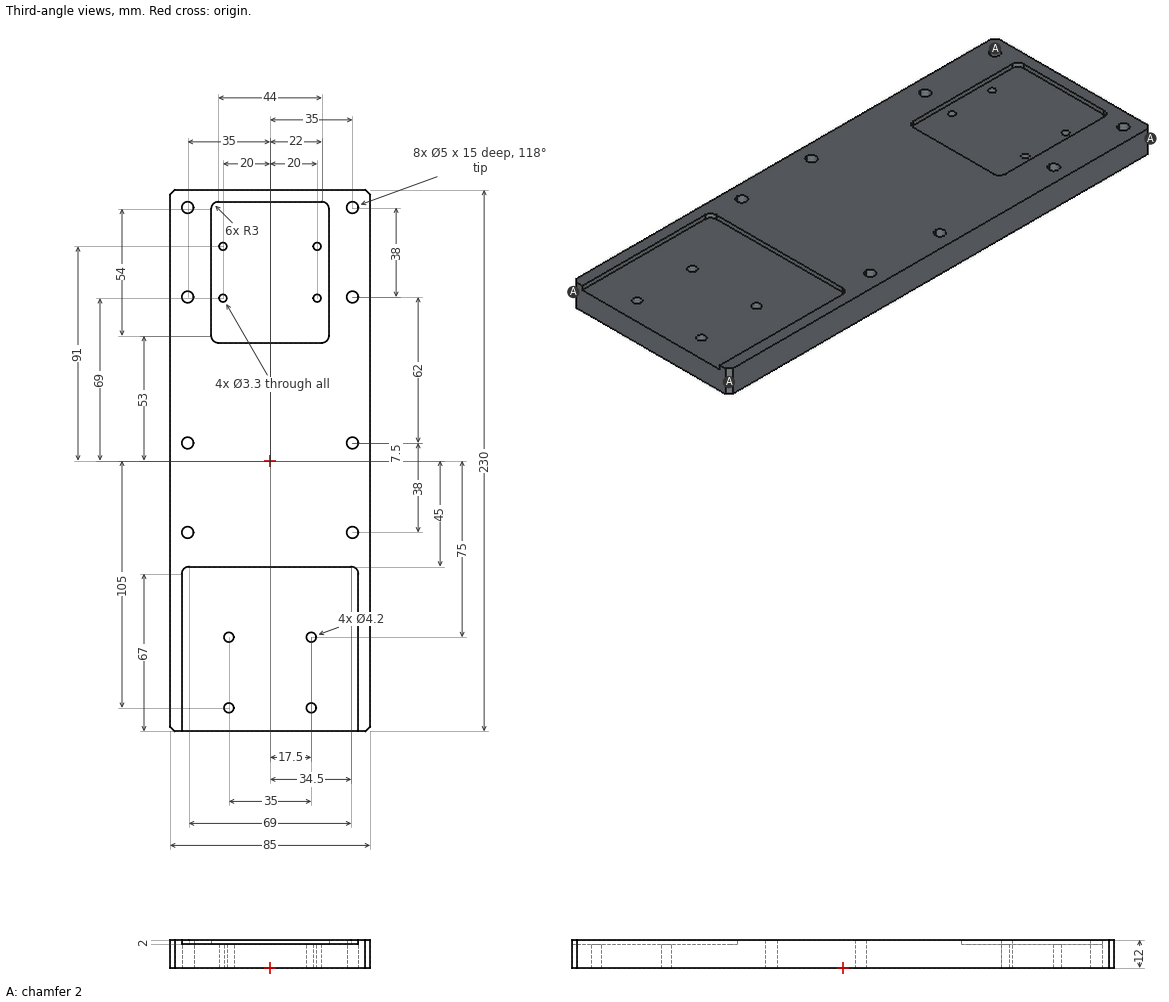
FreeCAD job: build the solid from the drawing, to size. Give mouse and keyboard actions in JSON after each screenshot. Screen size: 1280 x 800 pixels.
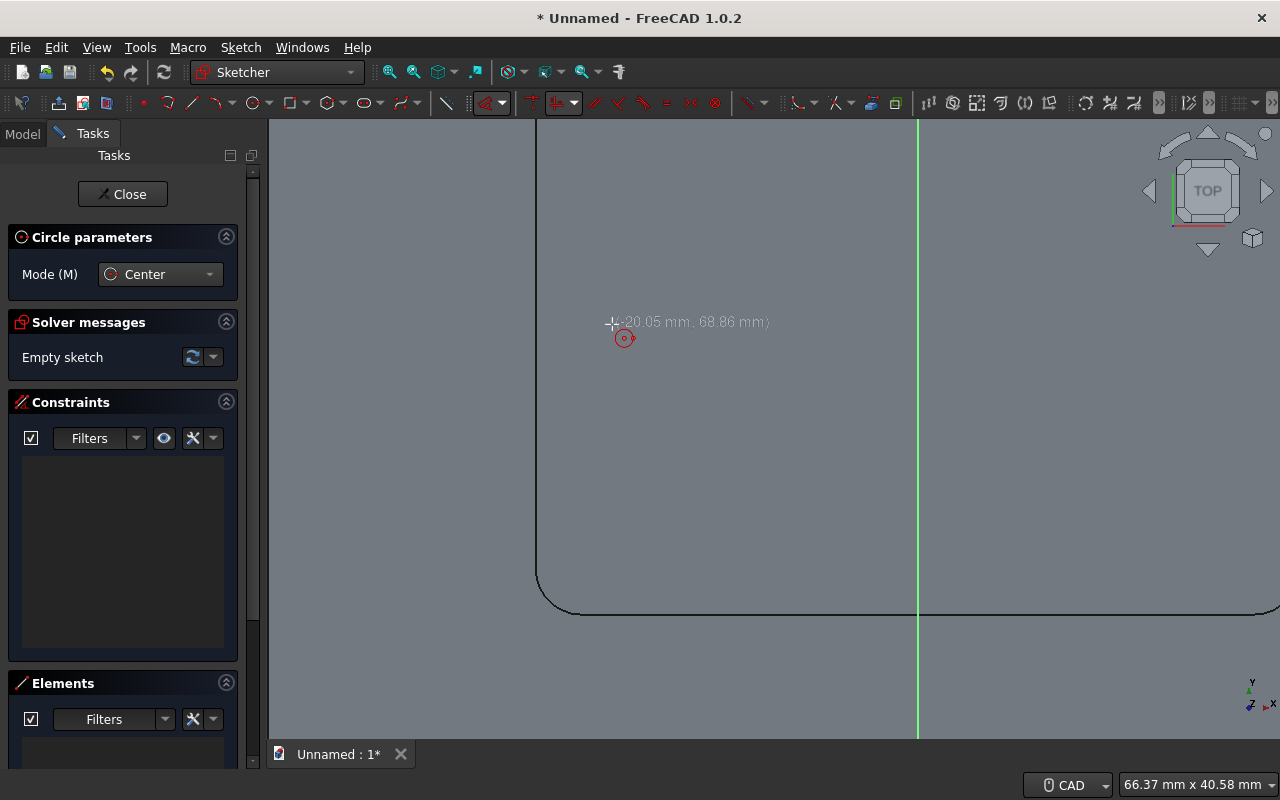
{"action": "left_click", "coordinate": [612, 324]}
{"action": "left_click", "coordinate": [630, 307]}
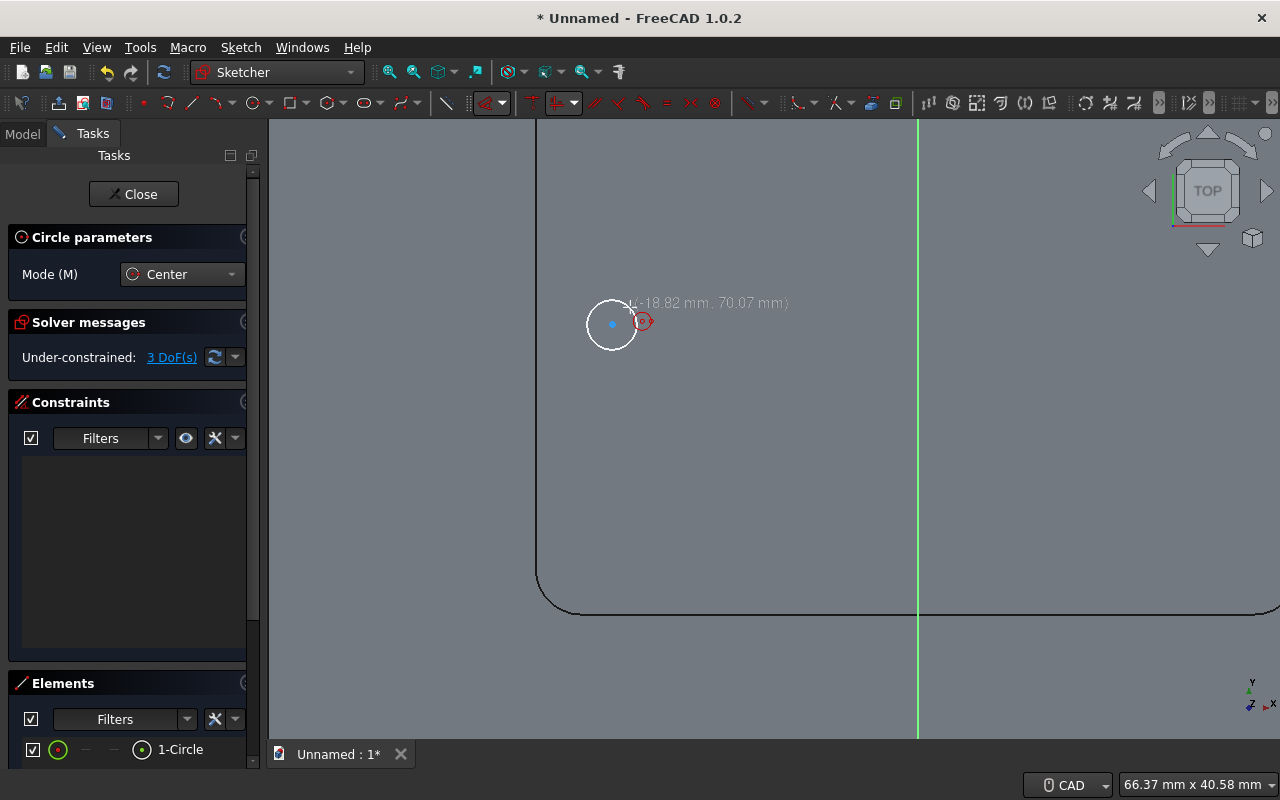
{"action": "scroll", "coordinate": [613, 325], "scroll_direction": "down", "scroll_amount": 6}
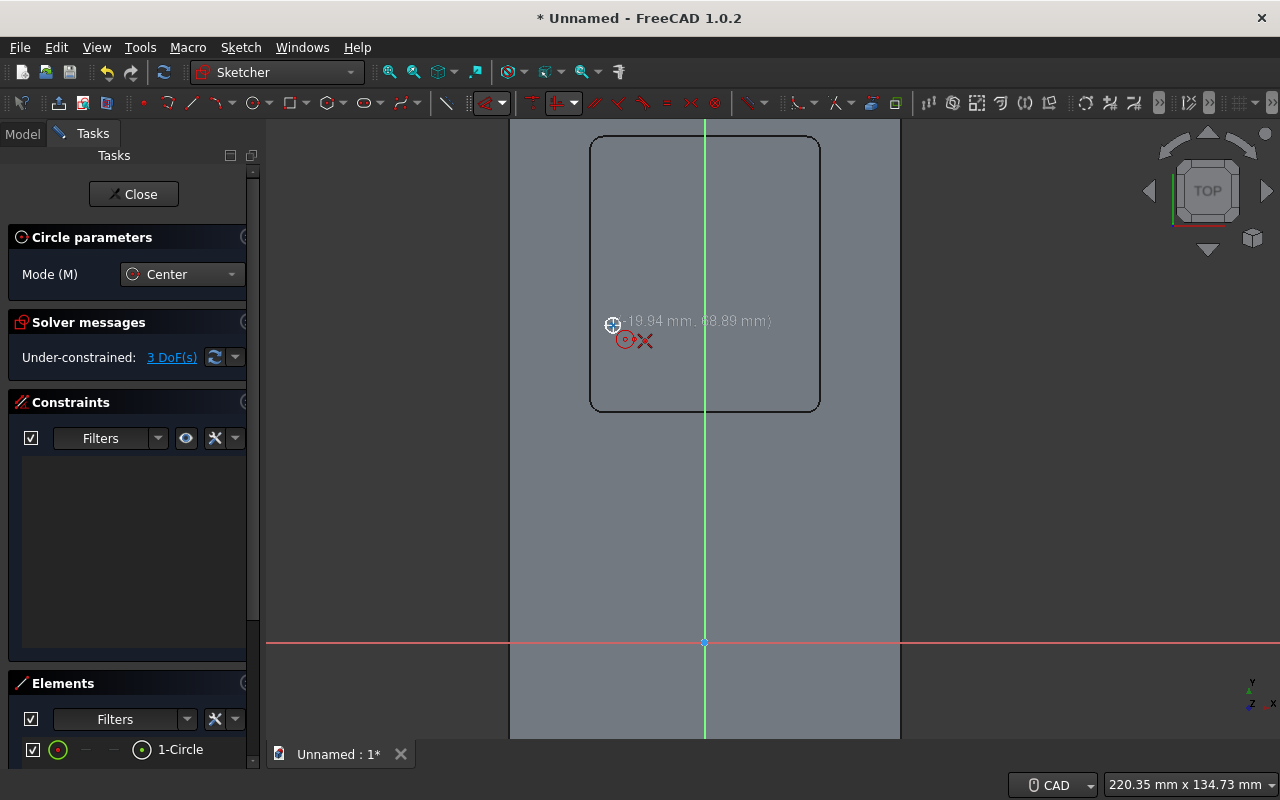
{"action": "scroll", "coordinate": [797, 325], "scroll_direction": "up", "scroll_amount": 6}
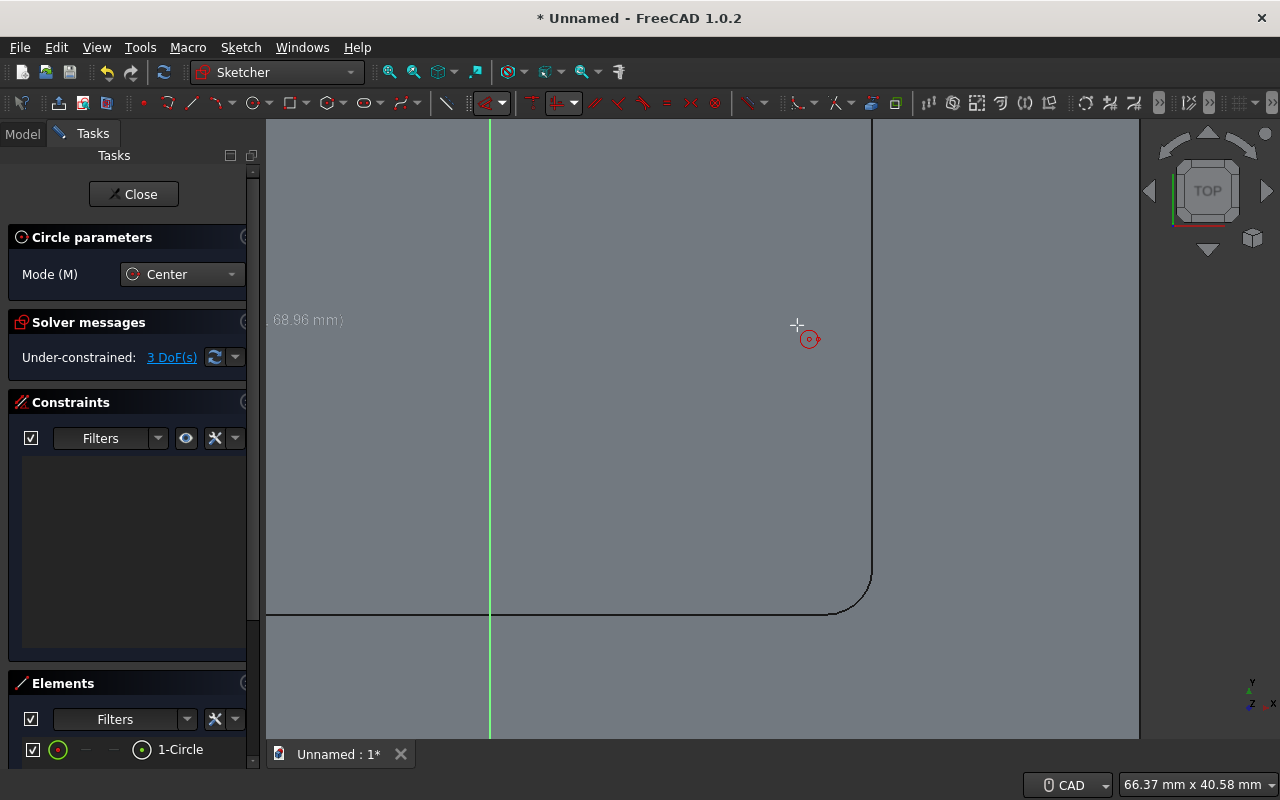
{"action": "left_click", "coordinate": [796, 324]}
{"action": "left_click", "coordinate": [814, 307]}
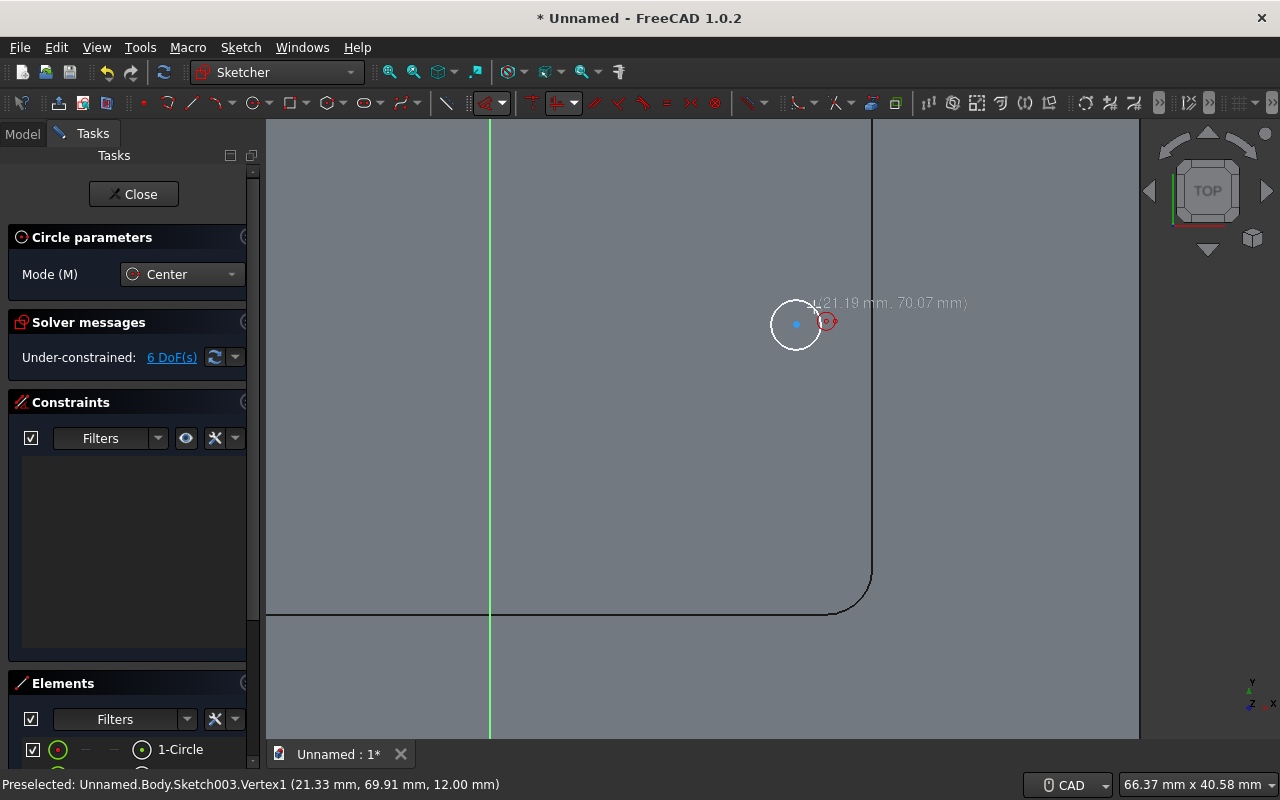
{"action": "scroll", "coordinate": [797, 325], "scroll_direction": "down", "scroll_amount": 6}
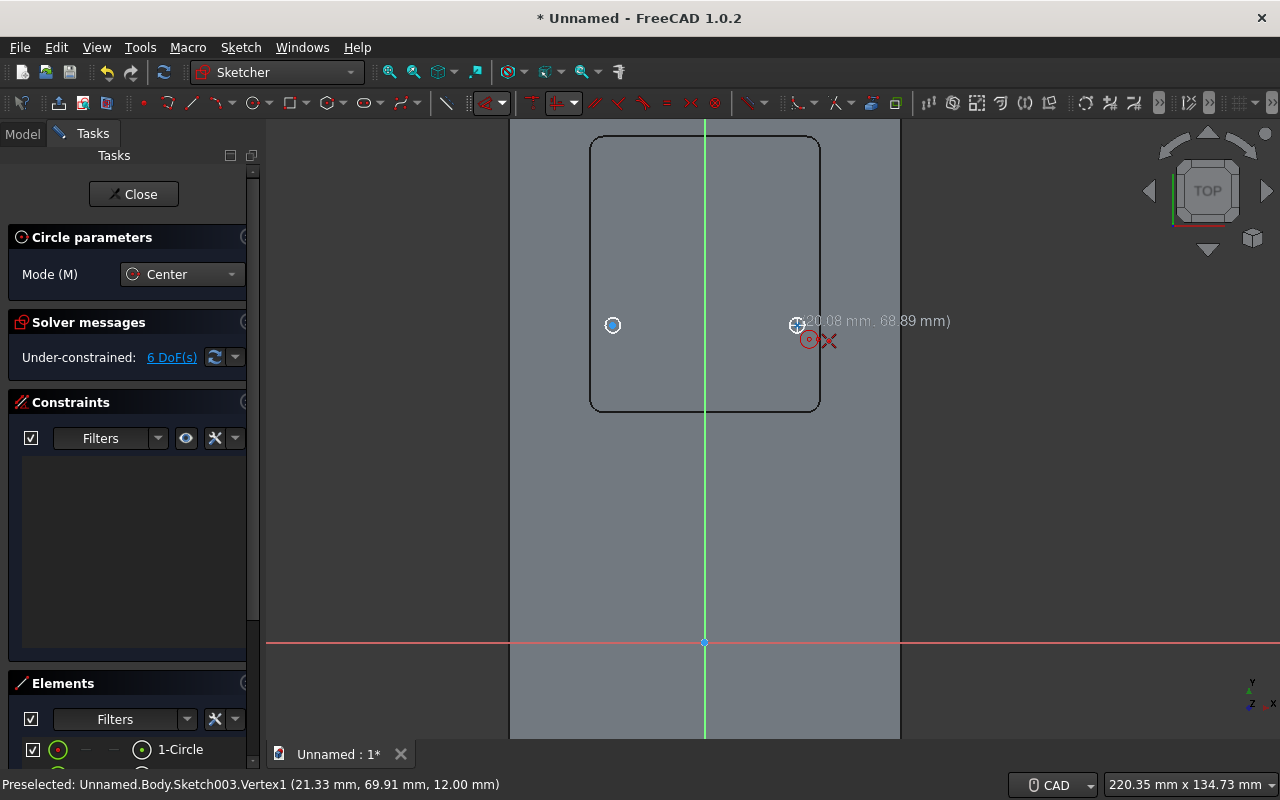
{"action": "scroll", "coordinate": [613, 224], "scroll_direction": "up", "scroll_amount": 6}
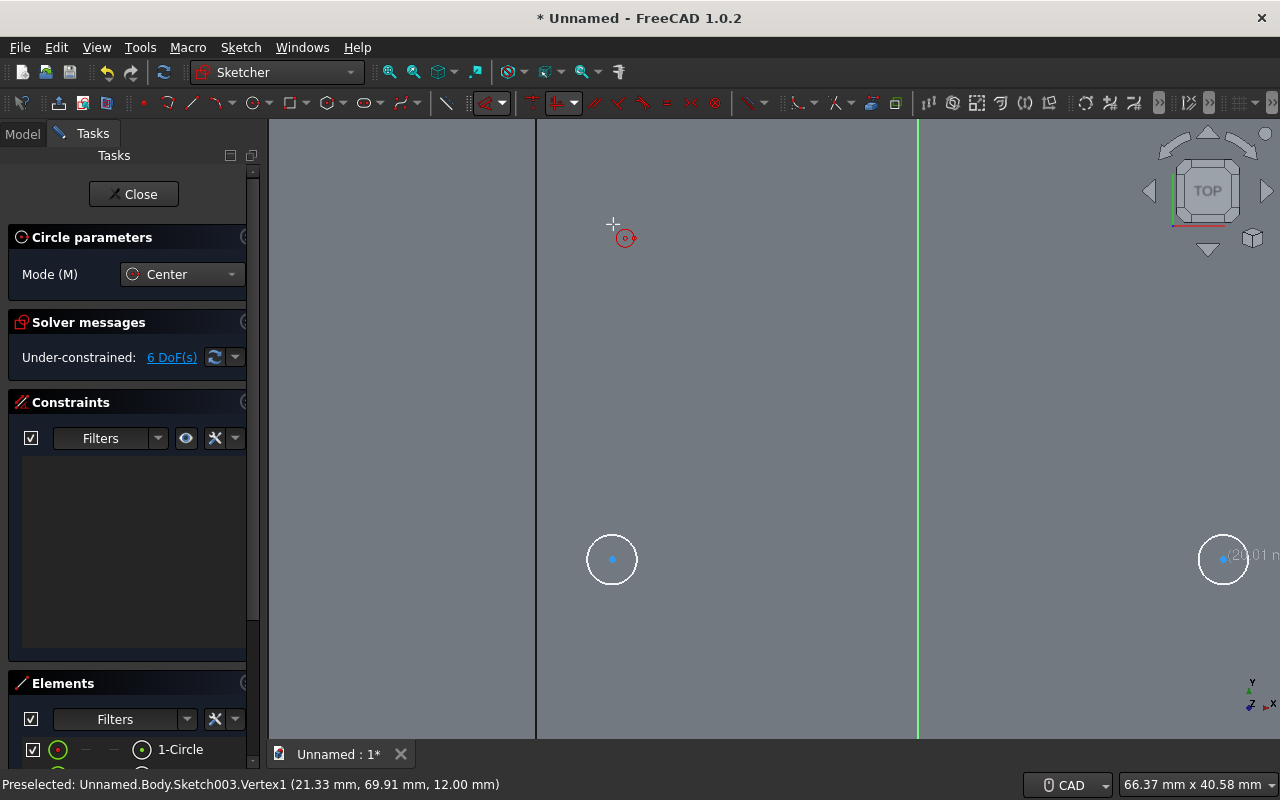
{"action": "left_click", "coordinate": [612, 223]}
{"action": "left_click", "coordinate": [630, 205]}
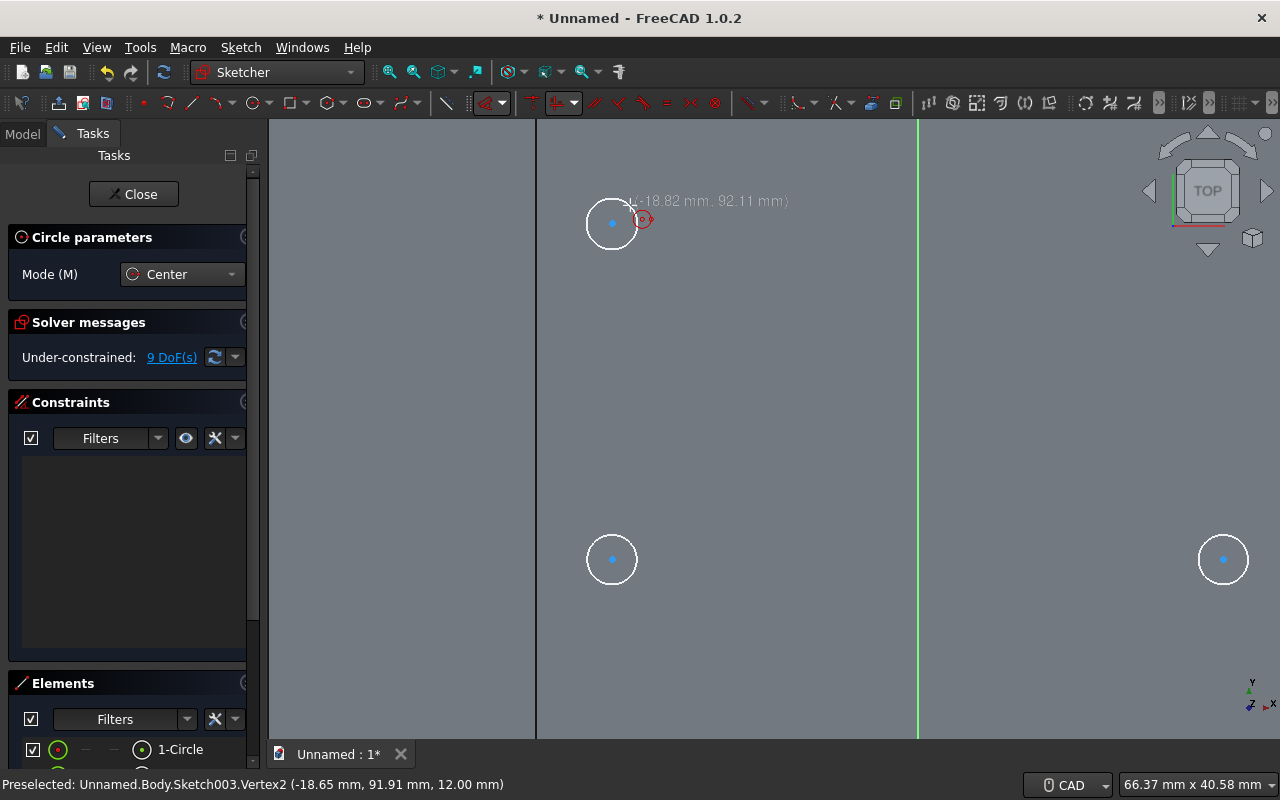
{"action": "scroll", "coordinate": [613, 224], "scroll_direction": "down", "scroll_amount": 6}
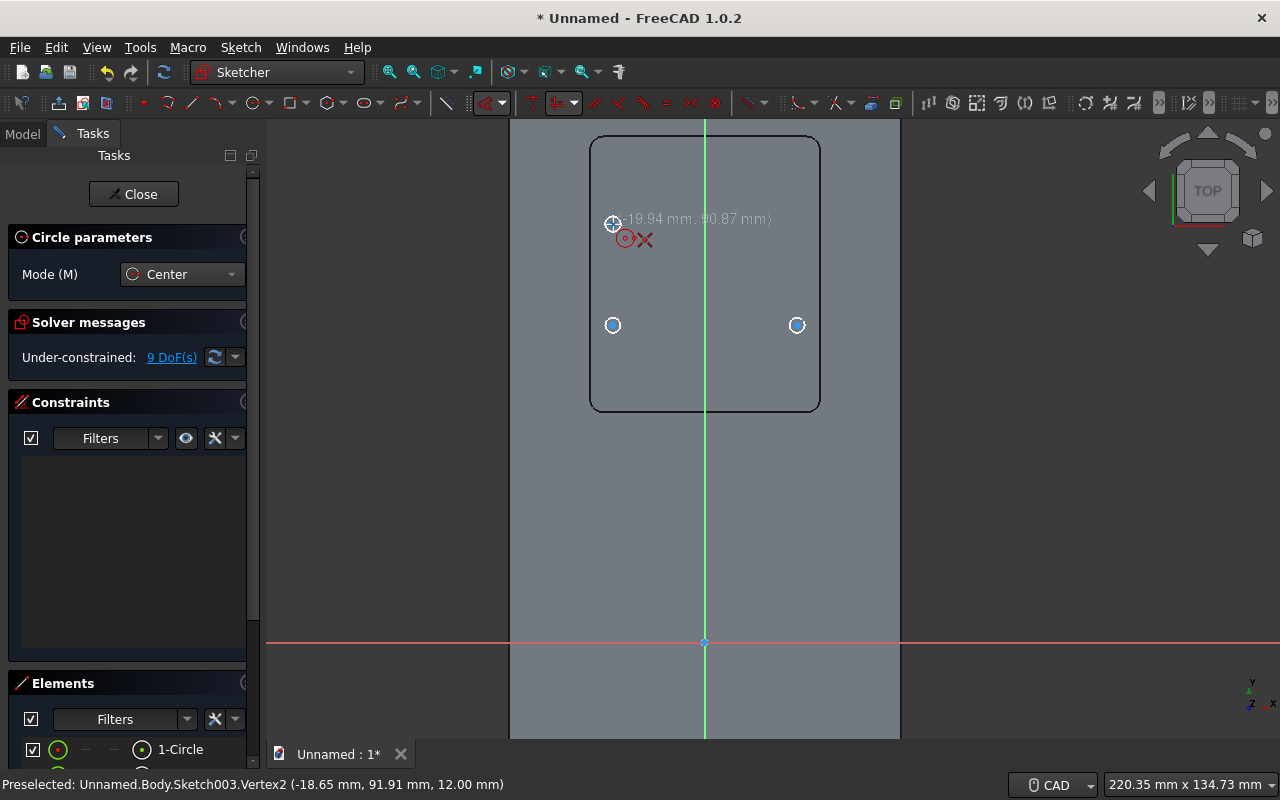
{"action": "scroll", "coordinate": [797, 224], "scroll_direction": "up", "scroll_amount": 6}